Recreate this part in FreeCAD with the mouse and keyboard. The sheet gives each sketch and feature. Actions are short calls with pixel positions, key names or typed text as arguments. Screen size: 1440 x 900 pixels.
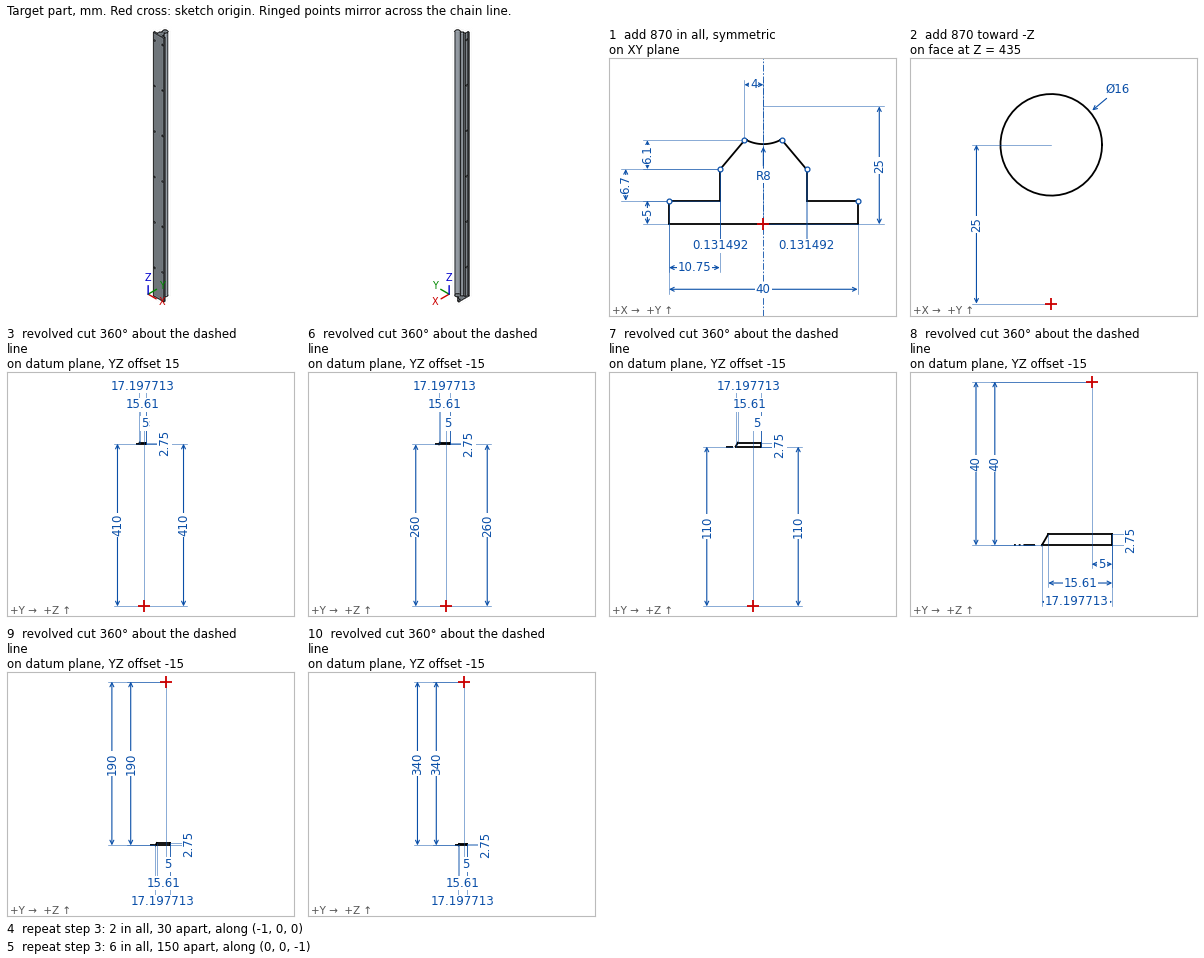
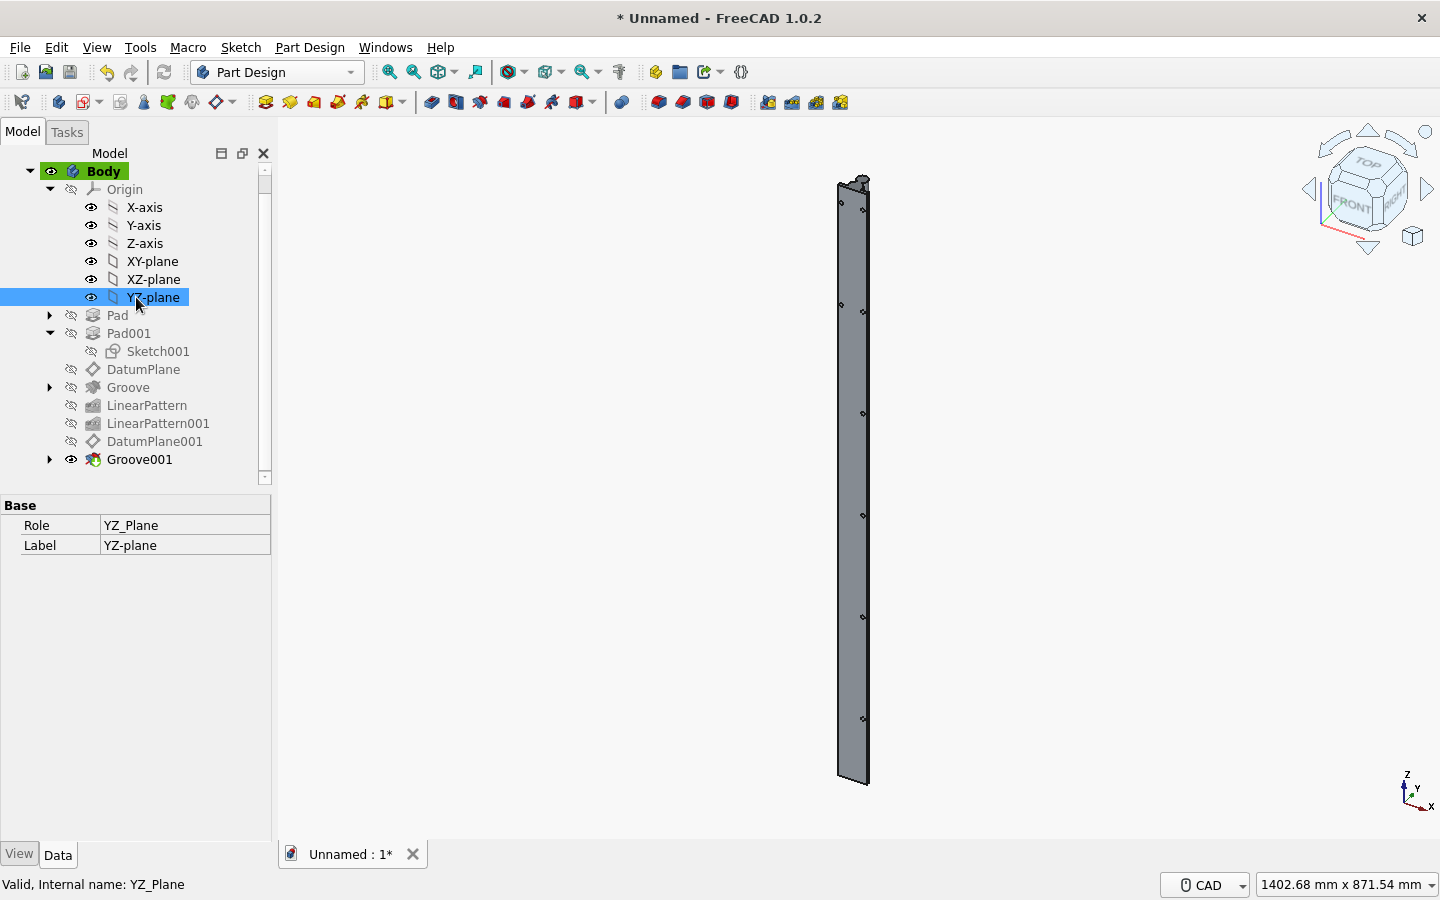
click(216, 102)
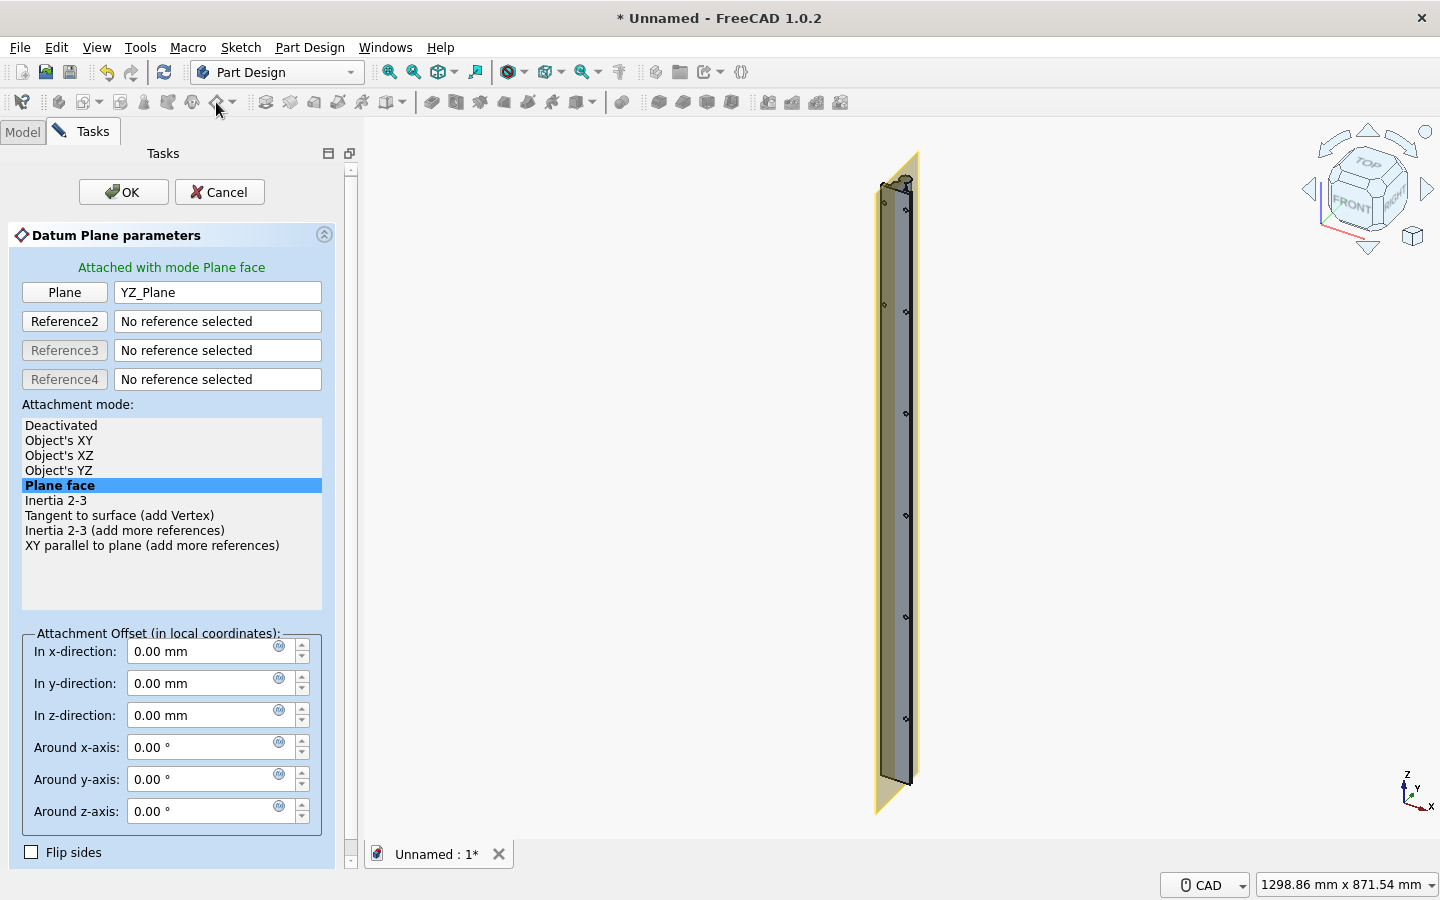
triple_click(210, 715)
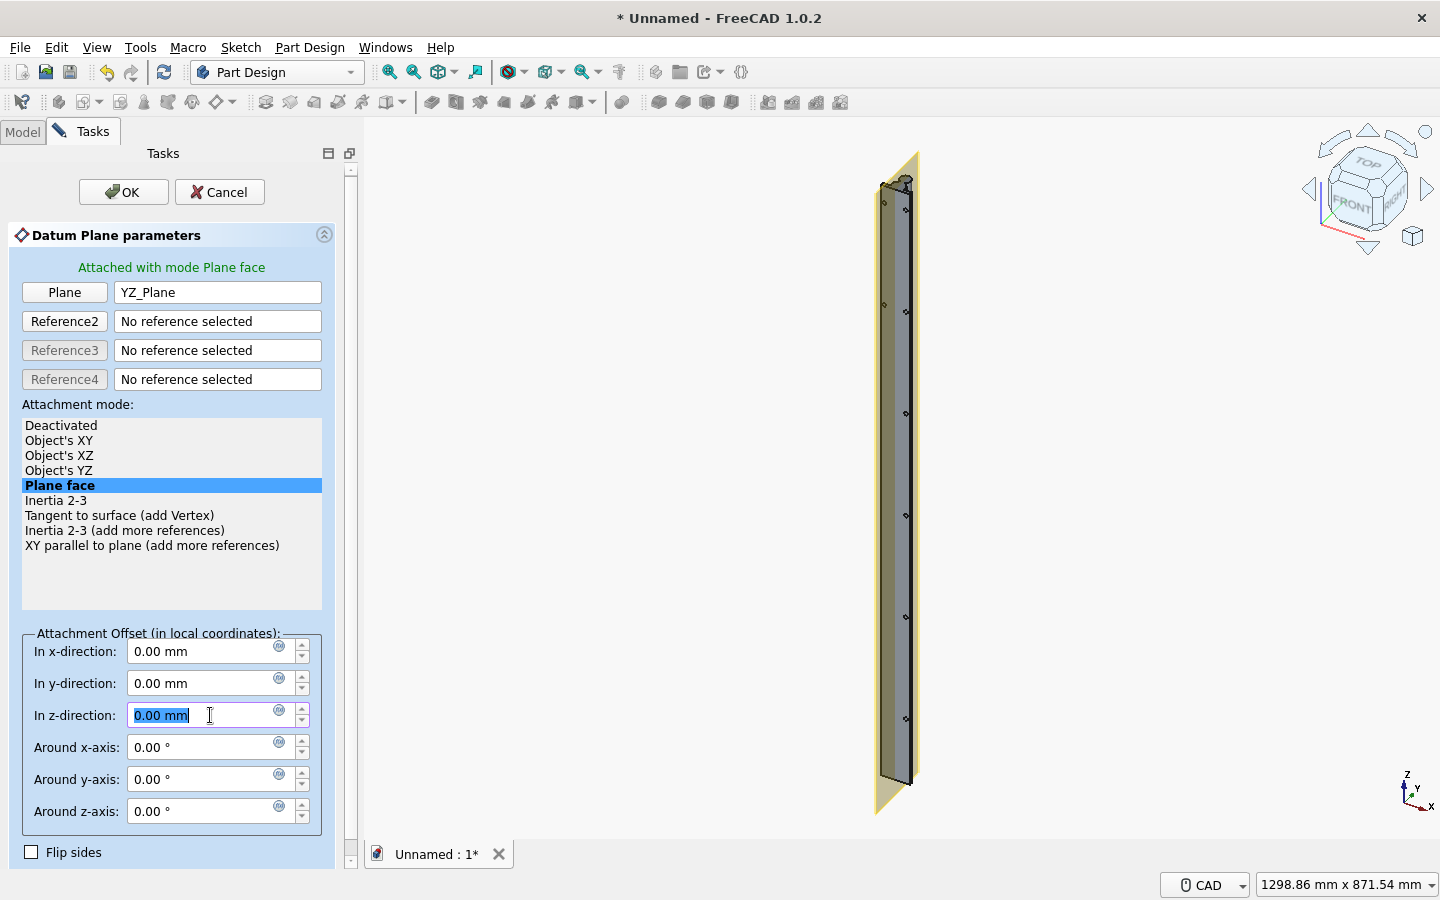
text(-15)
key(Tab)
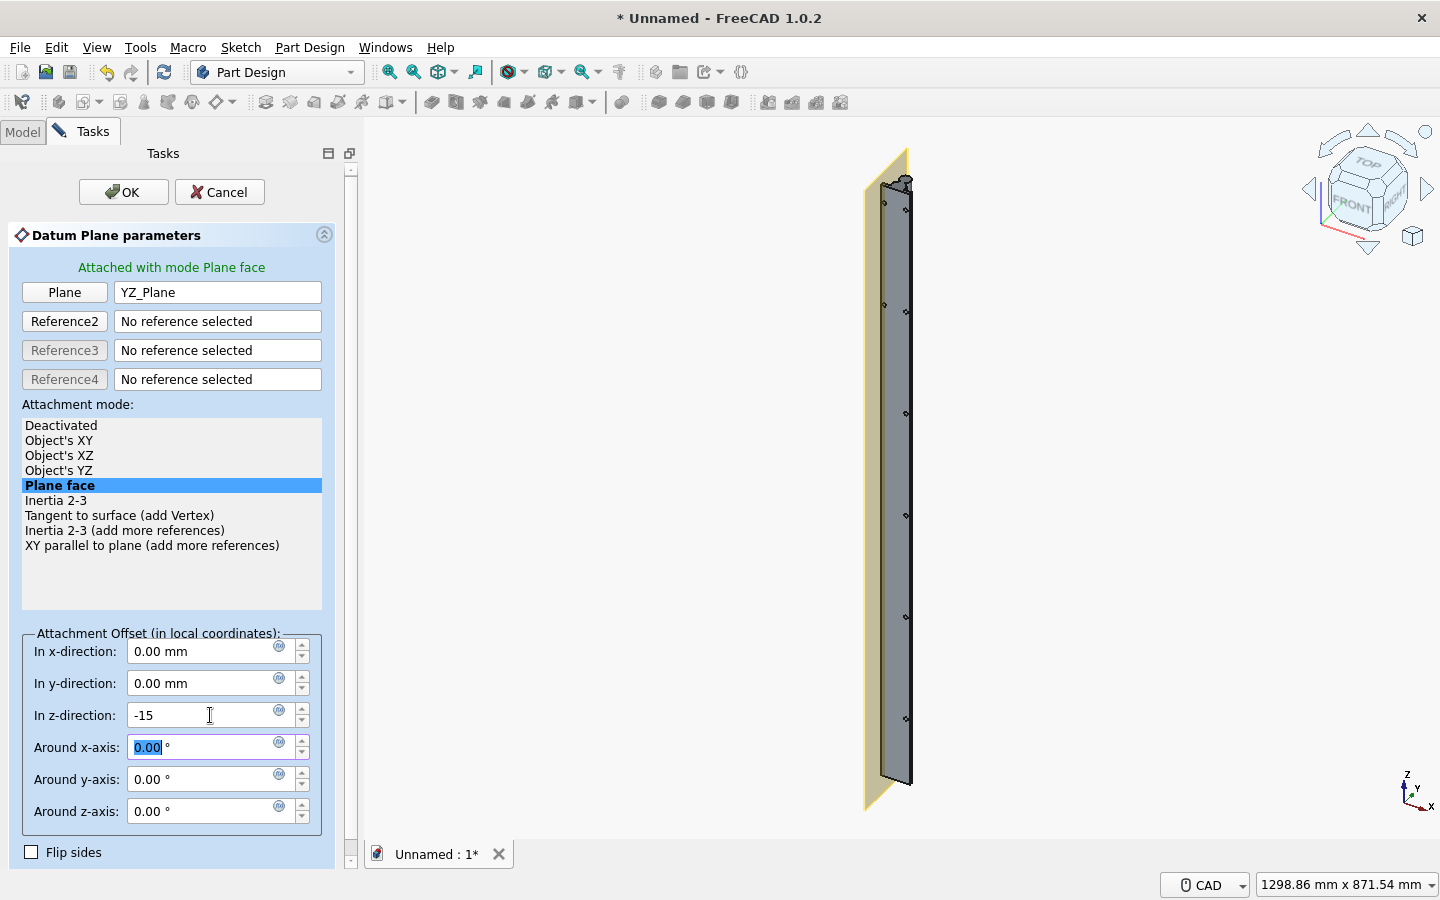
click(124, 192)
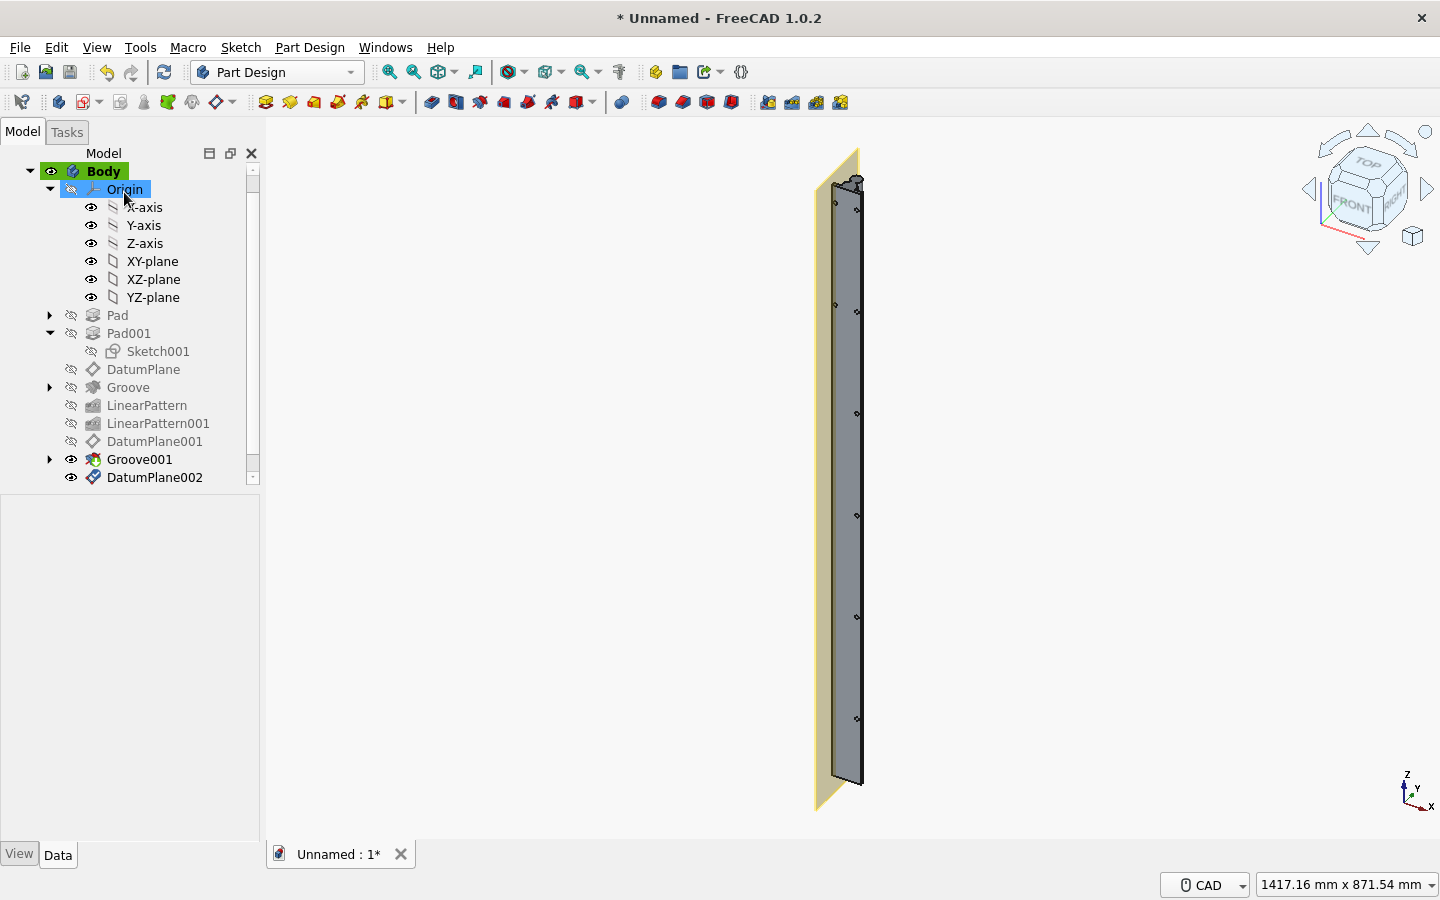
click(116, 477)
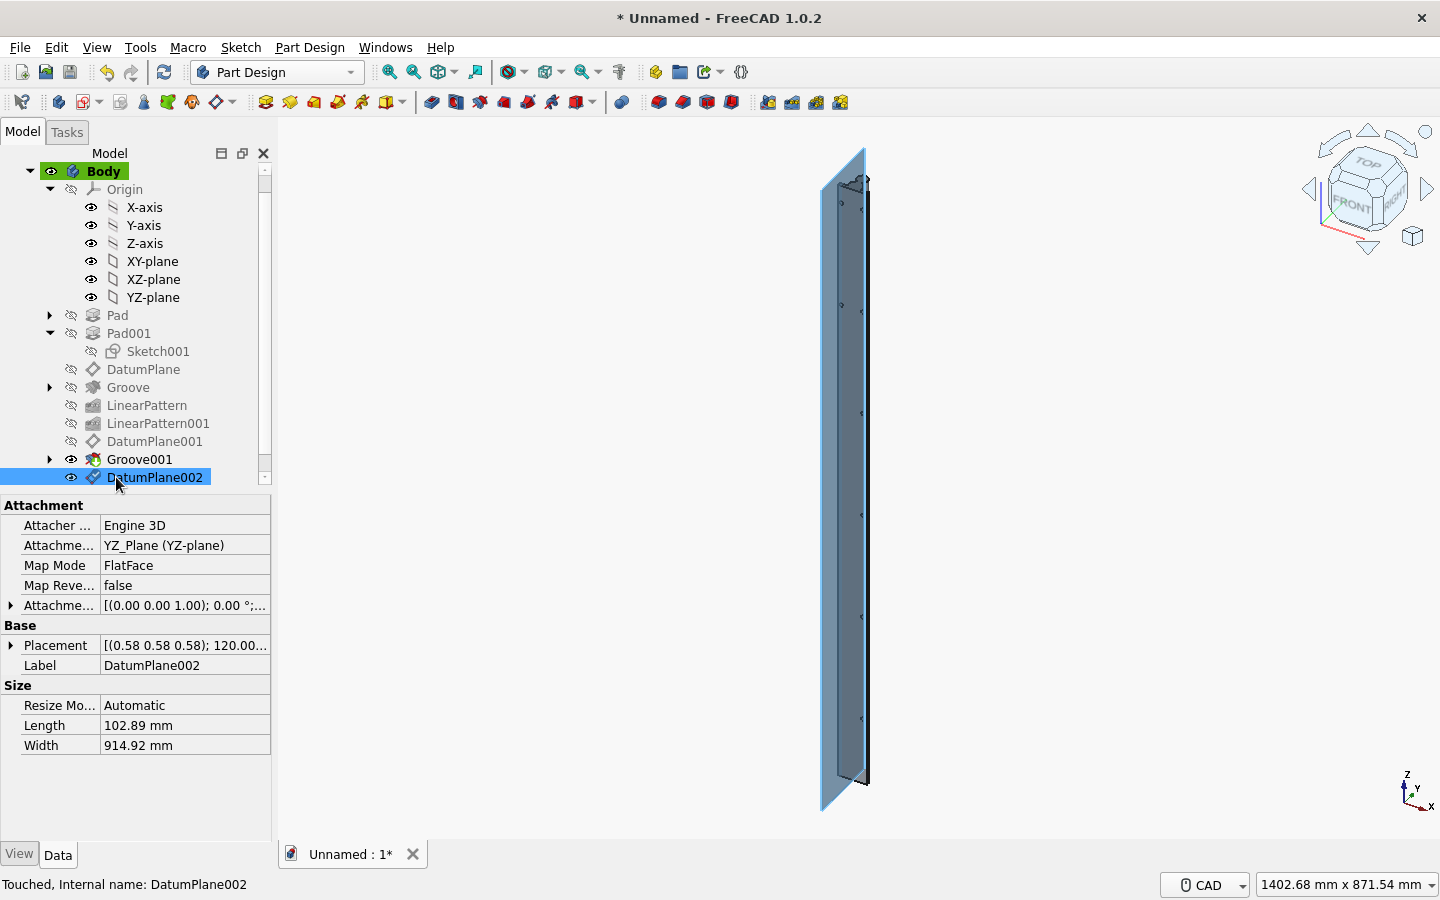
click(84, 102)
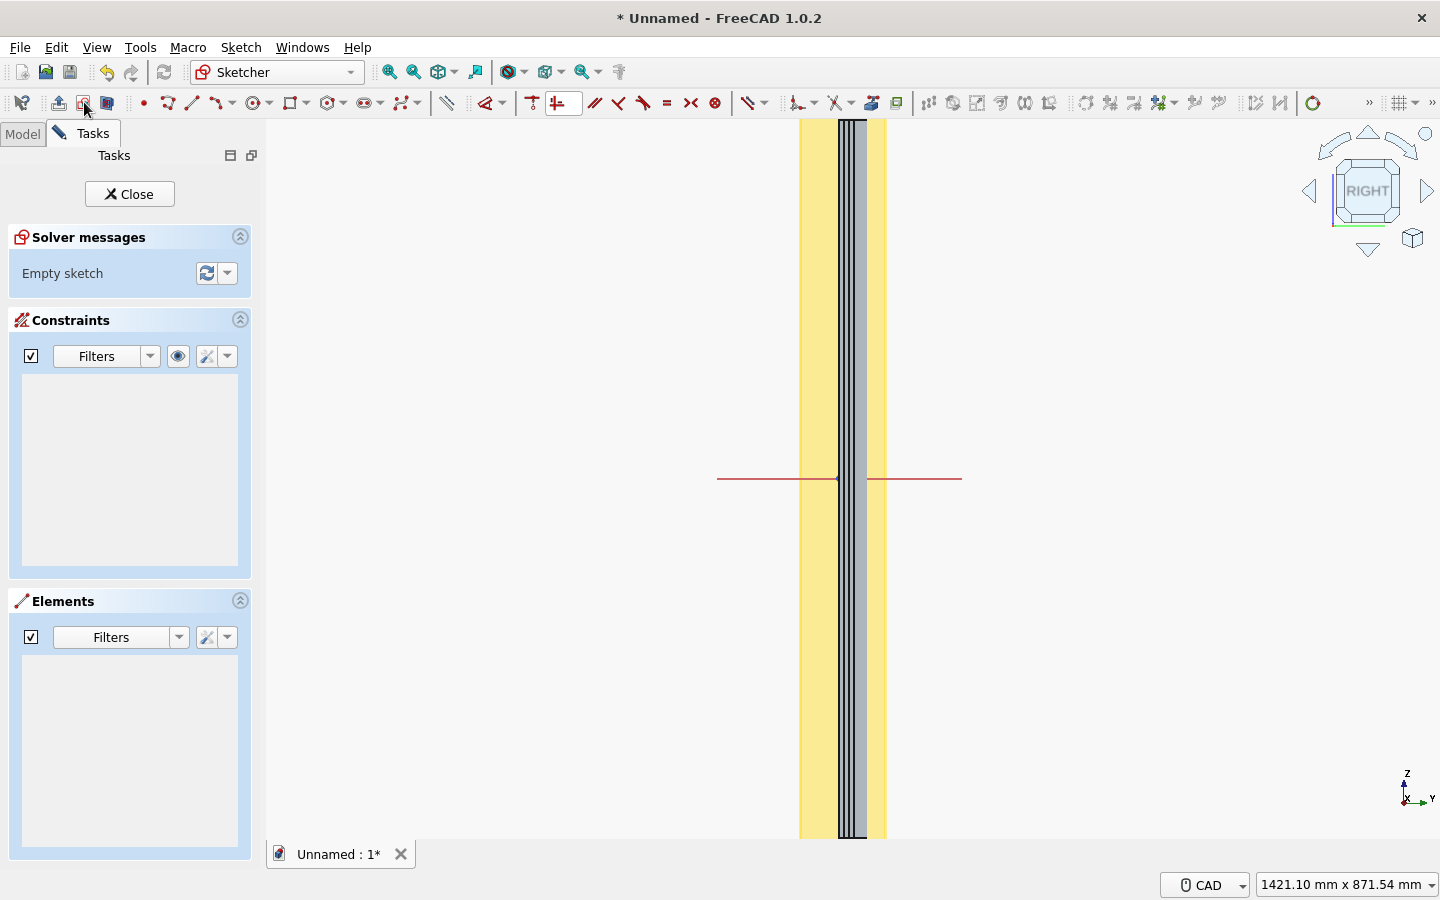
click(108, 104)